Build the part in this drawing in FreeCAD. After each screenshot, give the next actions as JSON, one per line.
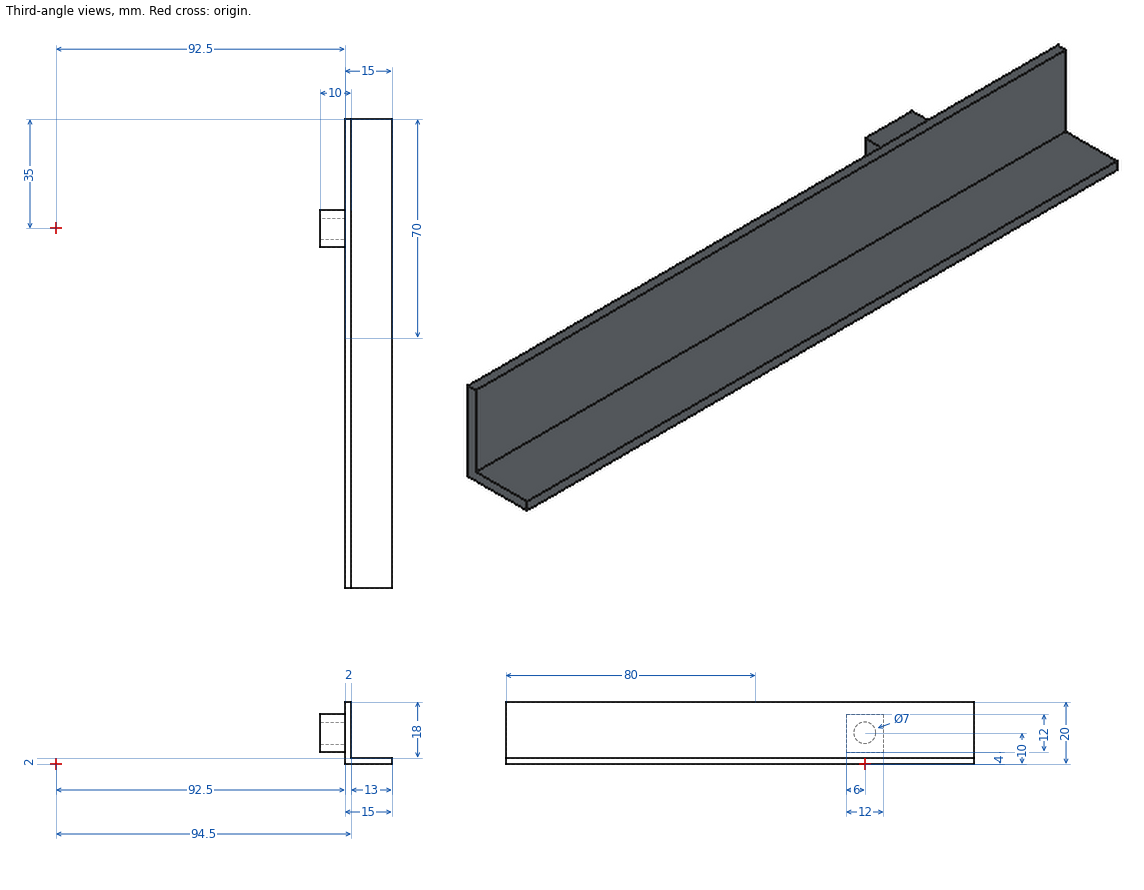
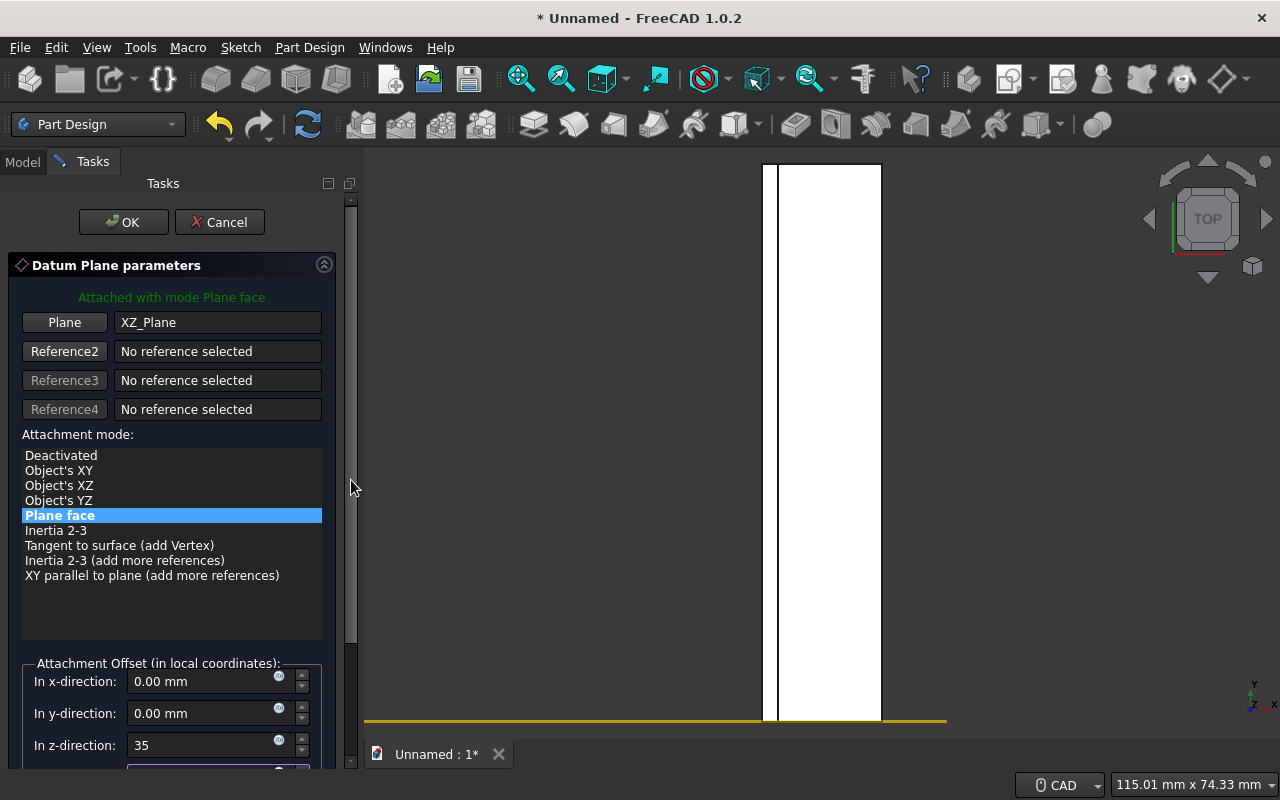
{"action": "left_click", "coordinate": [124, 222]}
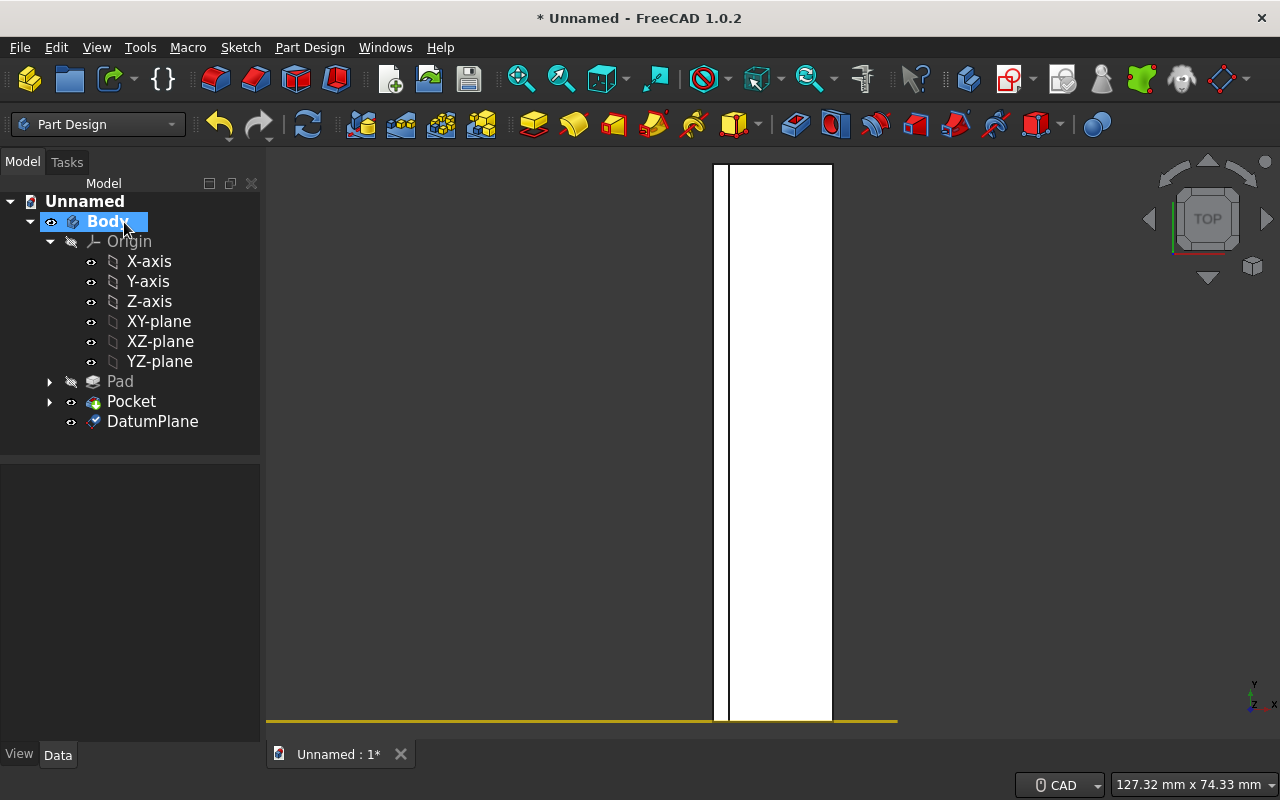
{"action": "left_click", "coordinate": [116, 422]}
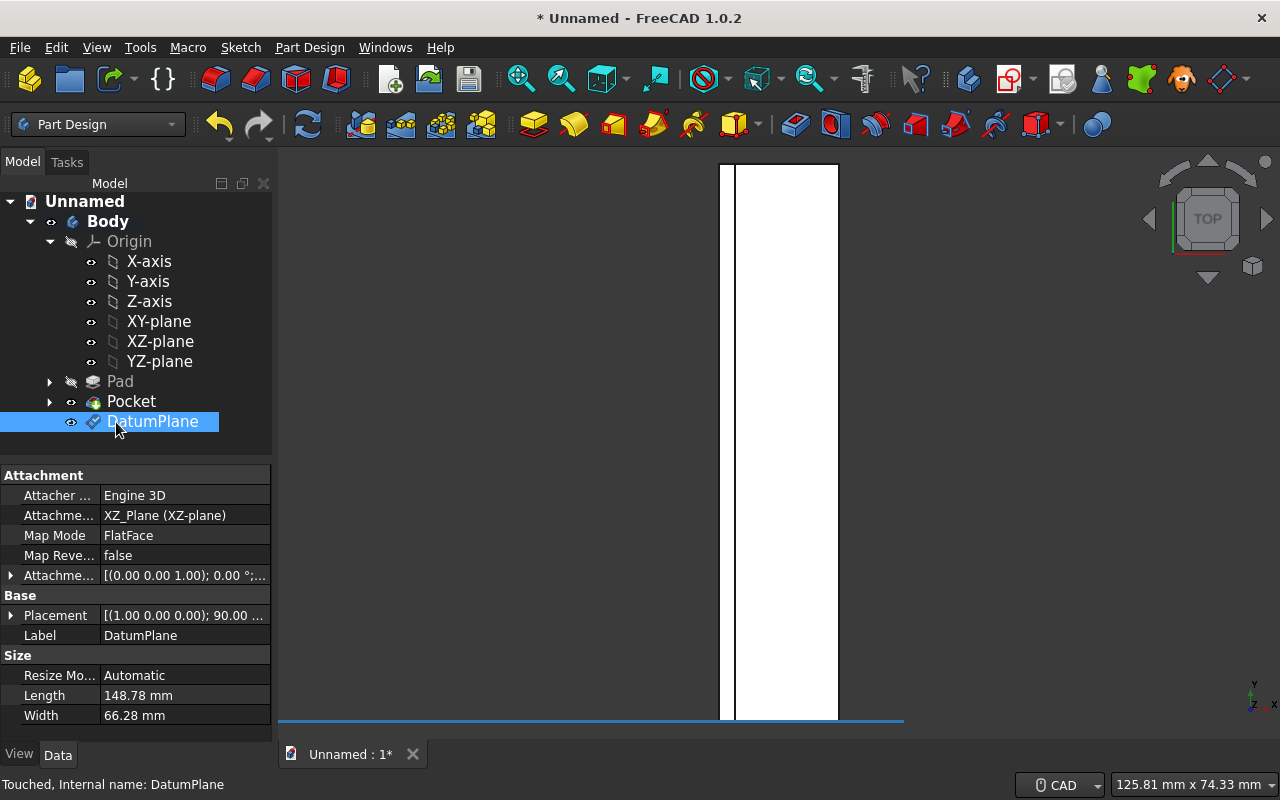
{"action": "left_click", "coordinate": [1010, 80]}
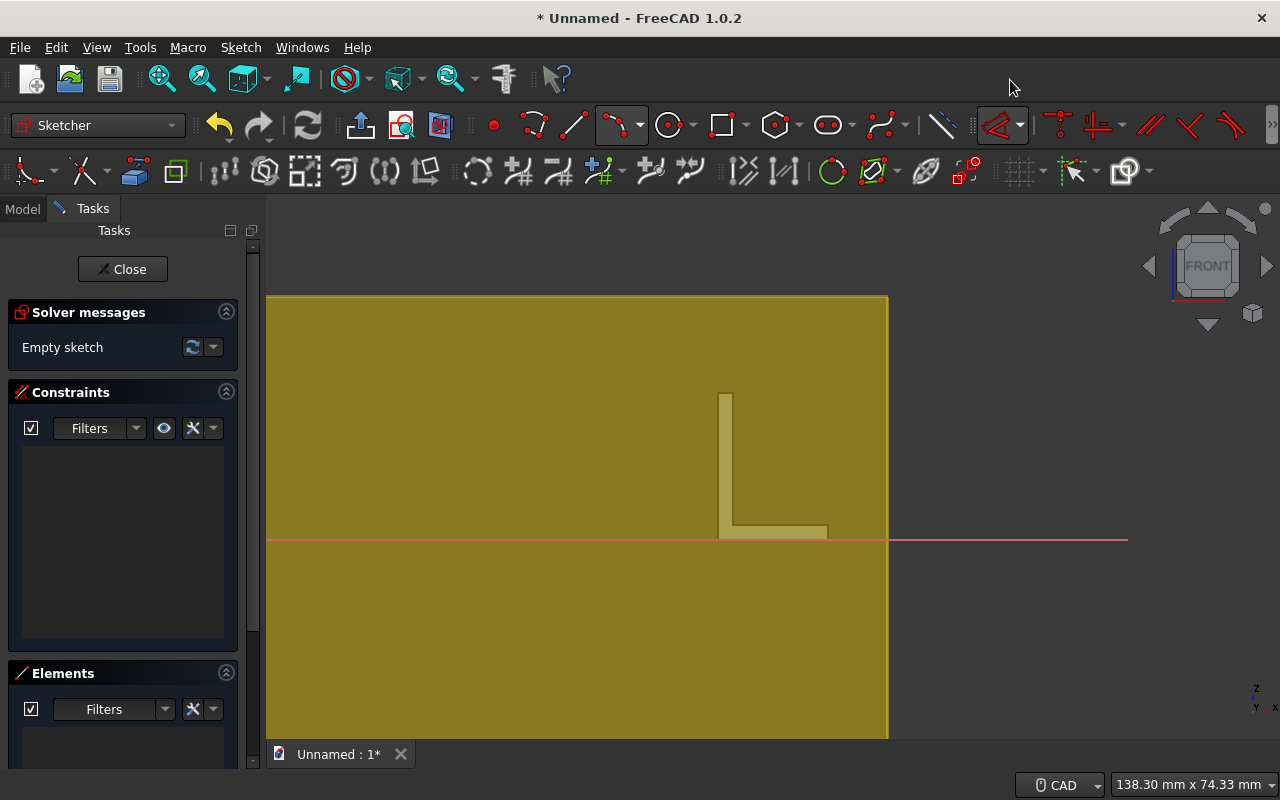
{"action": "scroll", "coordinate": [829, 466], "scroll_direction": "up", "scroll_amount": 4}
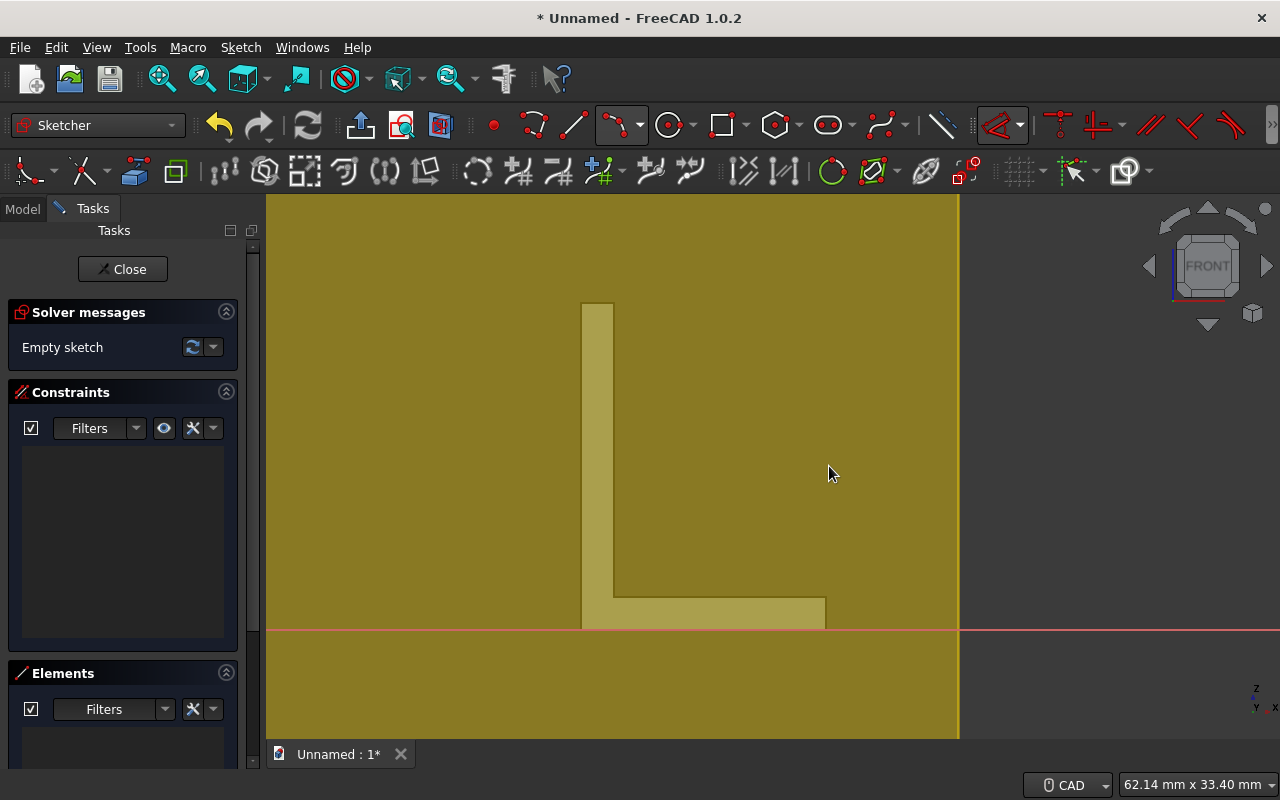
{"action": "left_click", "coordinate": [534, 126]}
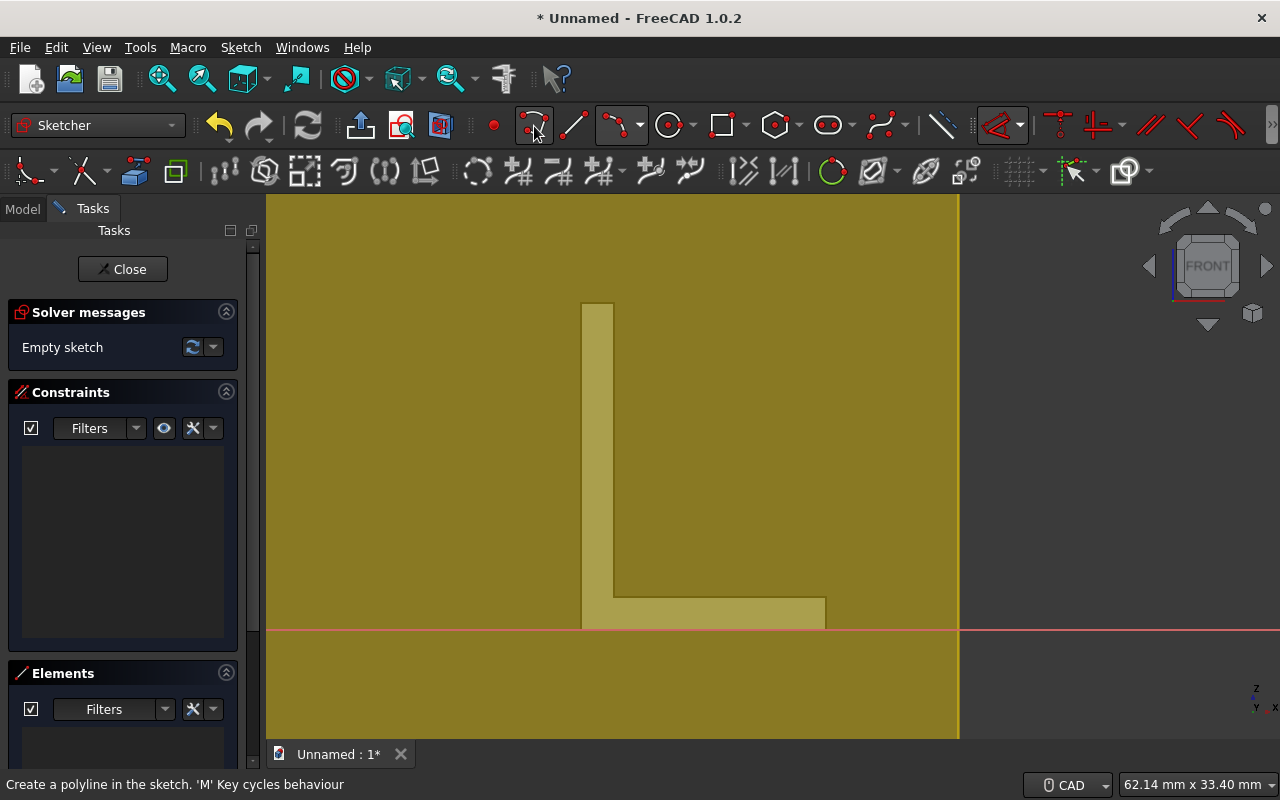
{"action": "left_click", "coordinate": [581, 630]}
{"action": "left_click", "coordinate": [826, 621]}
{"action": "left_click", "coordinate": [826, 597]}
{"action": "left_click", "coordinate": [614, 597]}
{"action": "left_click", "coordinate": [614, 303]}
{"action": "left_click", "coordinate": [581, 303]}
{"action": "left_click", "coordinate": [581, 630]}
{"action": "key", "text": "Escape"}
{"action": "key", "text": "Escape"}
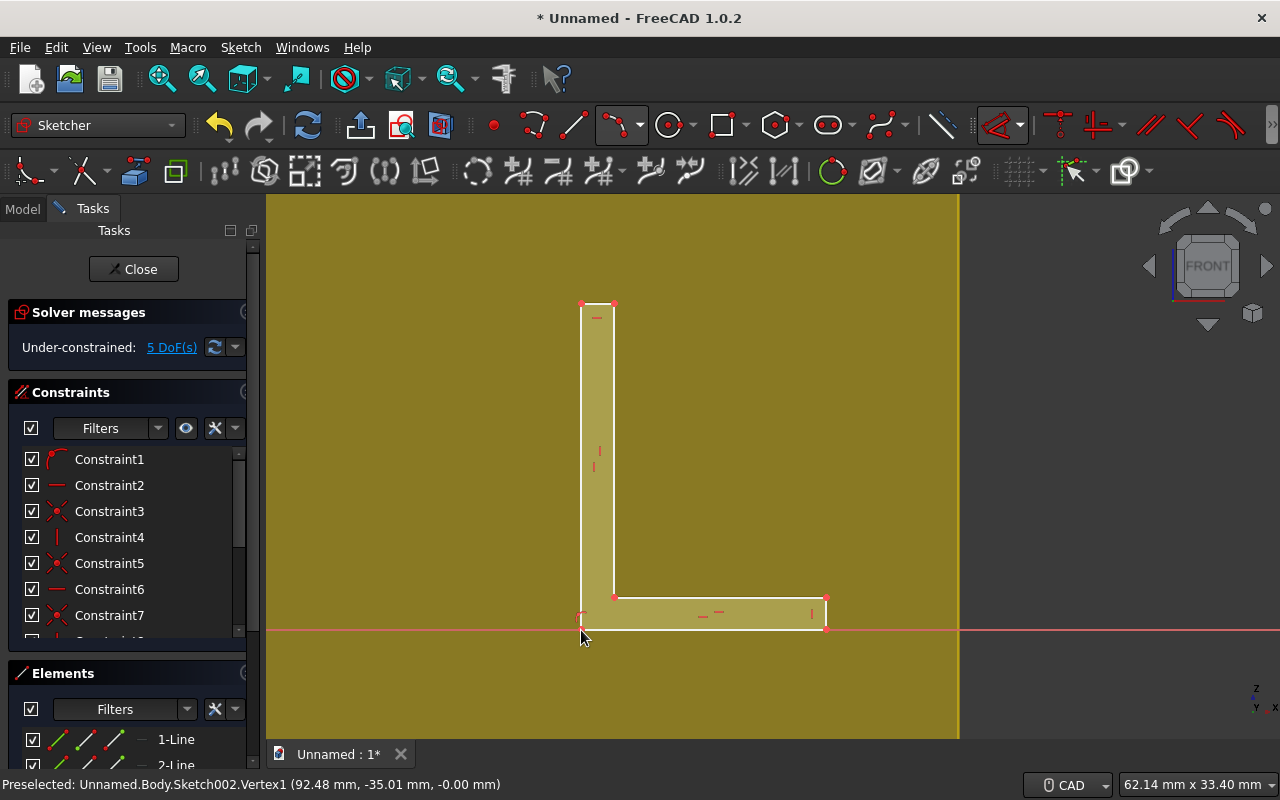
{"action": "scroll", "coordinate": [826, 620], "scroll_direction": "up", "scroll_amount": 2}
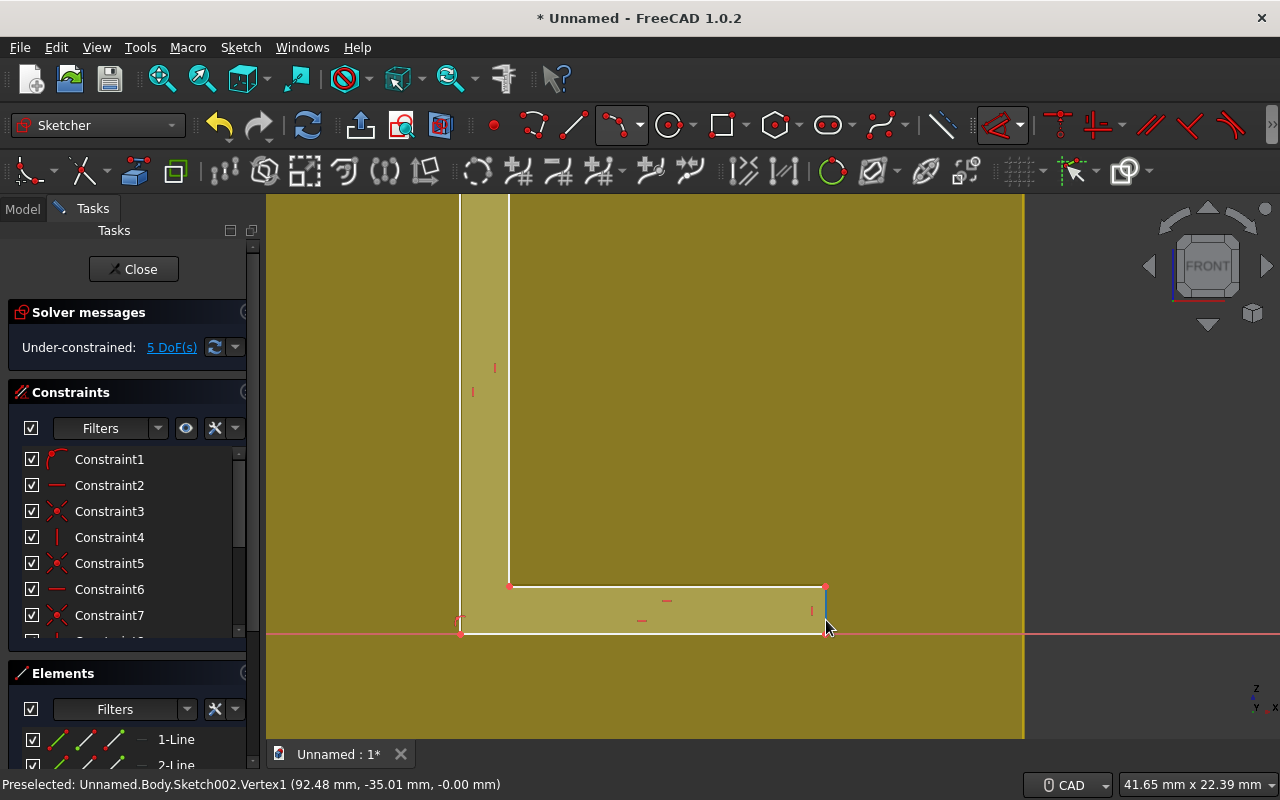
{"action": "left_click", "coordinate": [826, 620]}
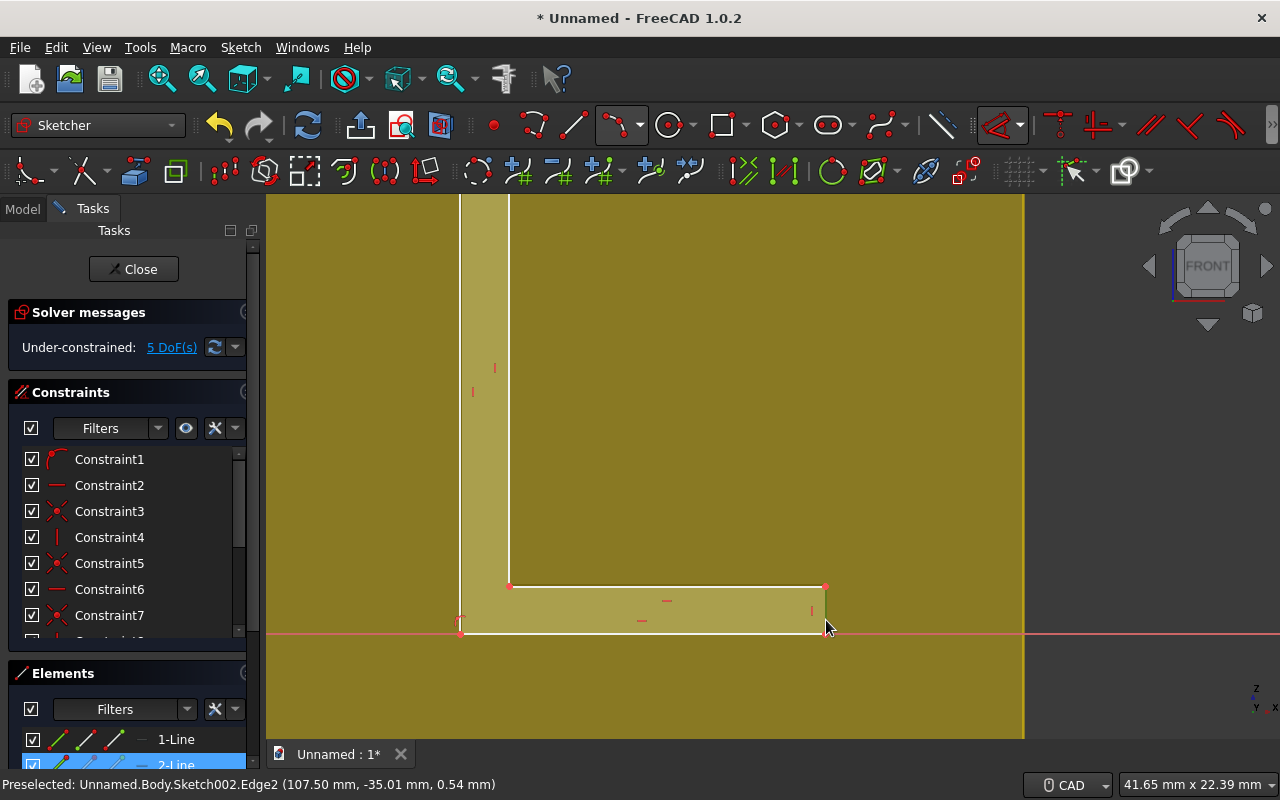
{"action": "left_click", "coordinate": [1022, 126]}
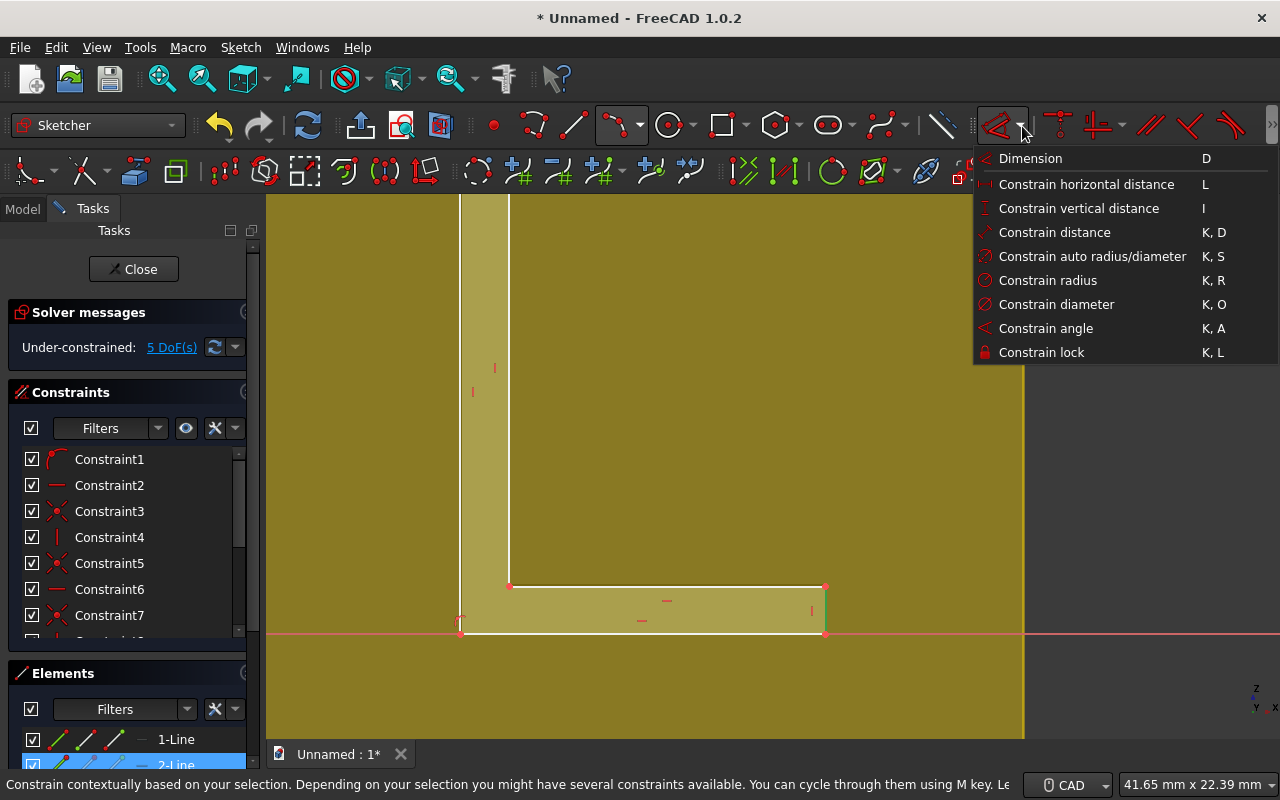
{"action": "left_click", "coordinate": [1126, 208]}